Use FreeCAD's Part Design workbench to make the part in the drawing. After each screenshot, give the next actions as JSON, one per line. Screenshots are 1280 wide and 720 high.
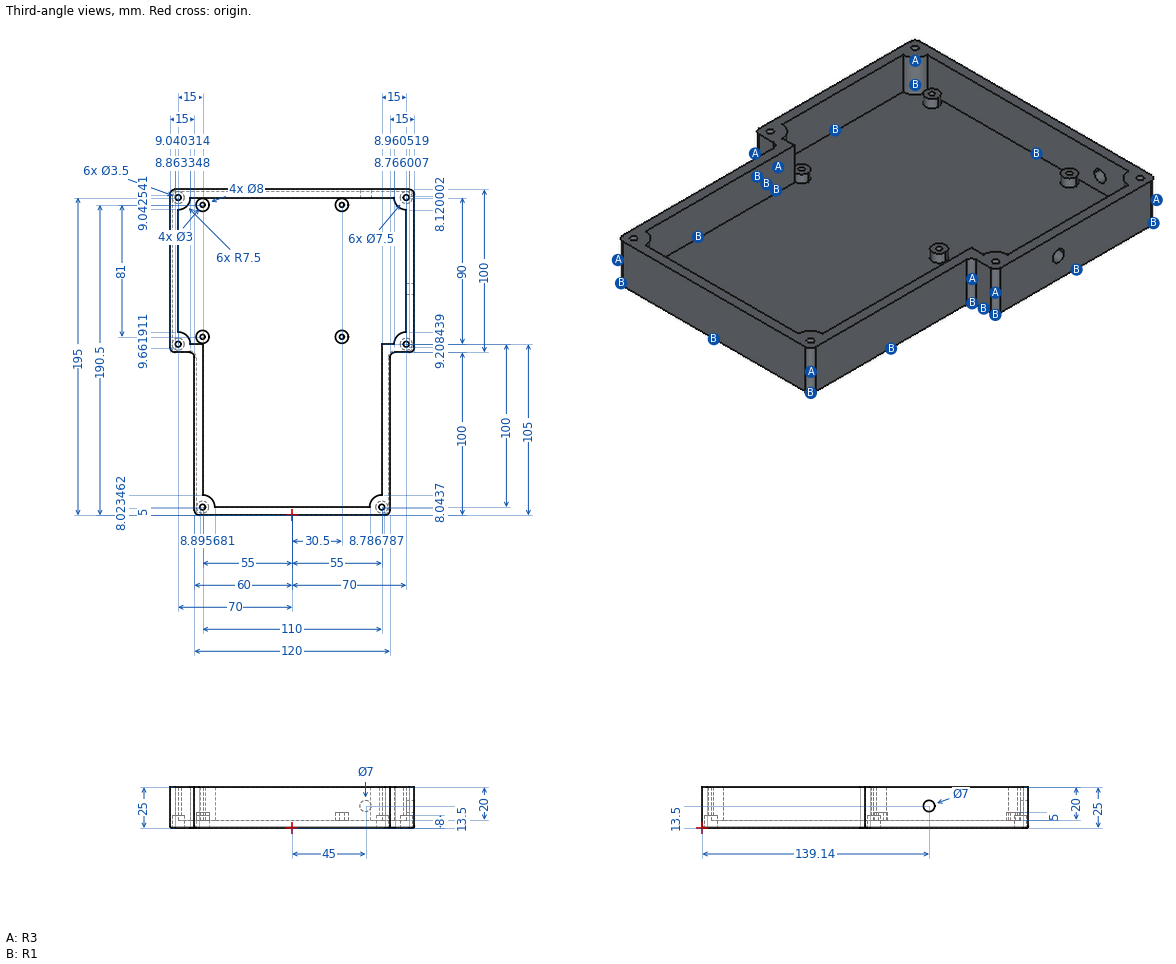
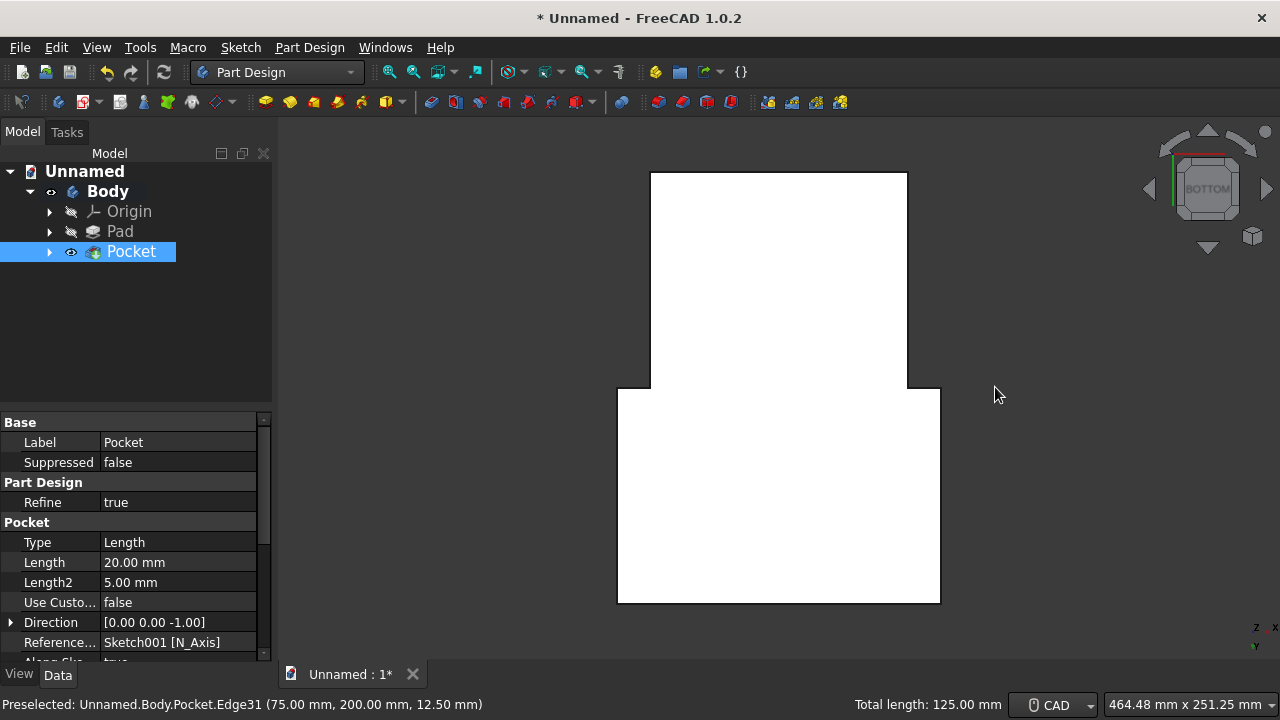
{"action": "key", "text": "4"}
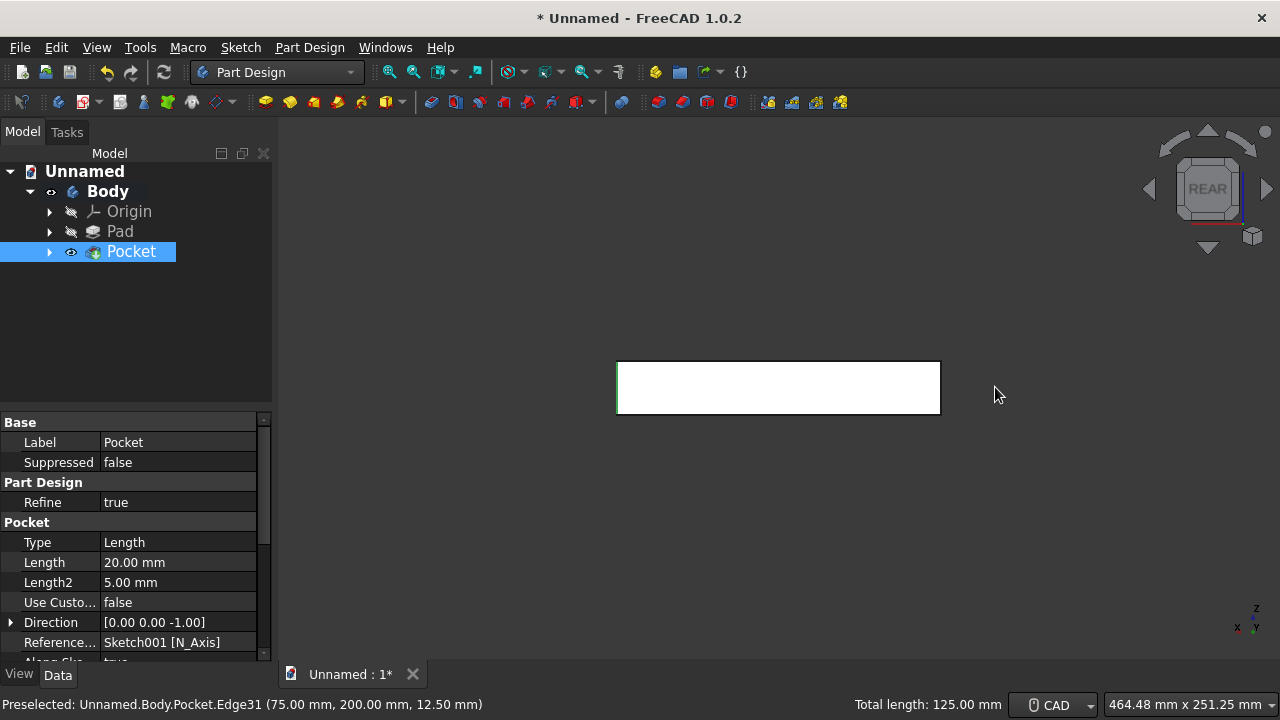
{"action": "key", "text": "v f"}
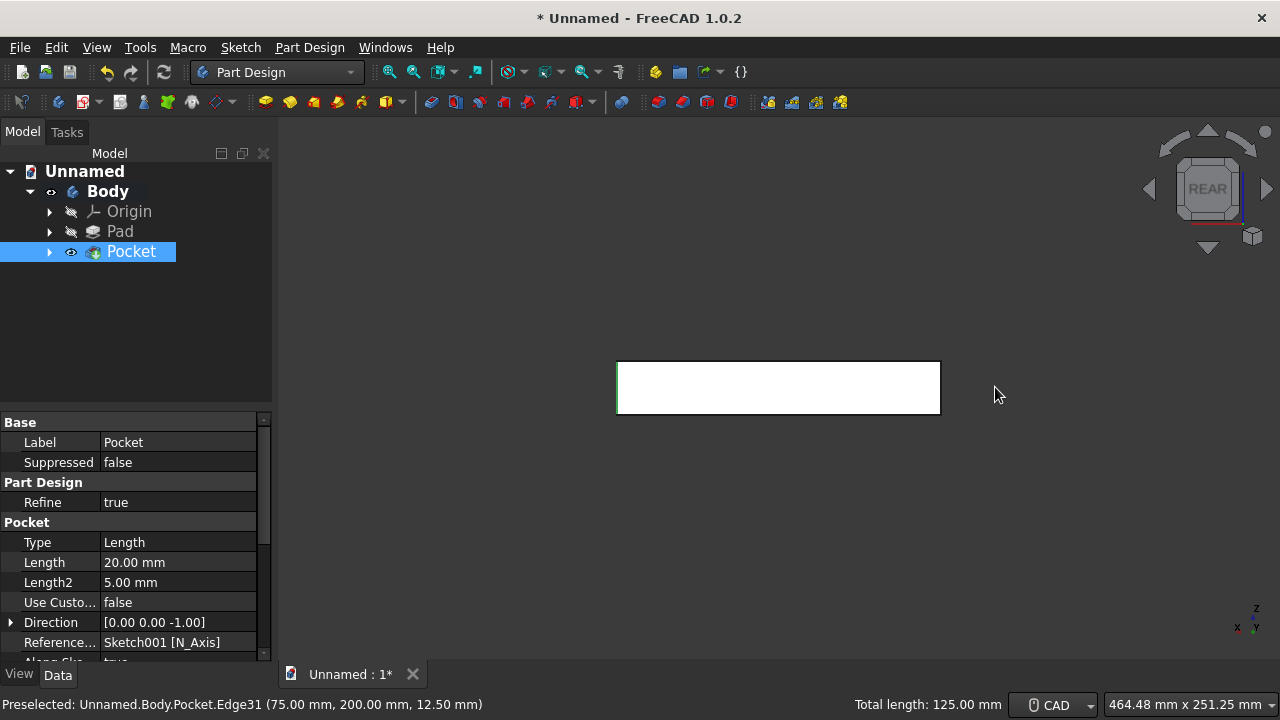
{"action": "left_click", "coordinate": [941, 387], "text": "ctrl"}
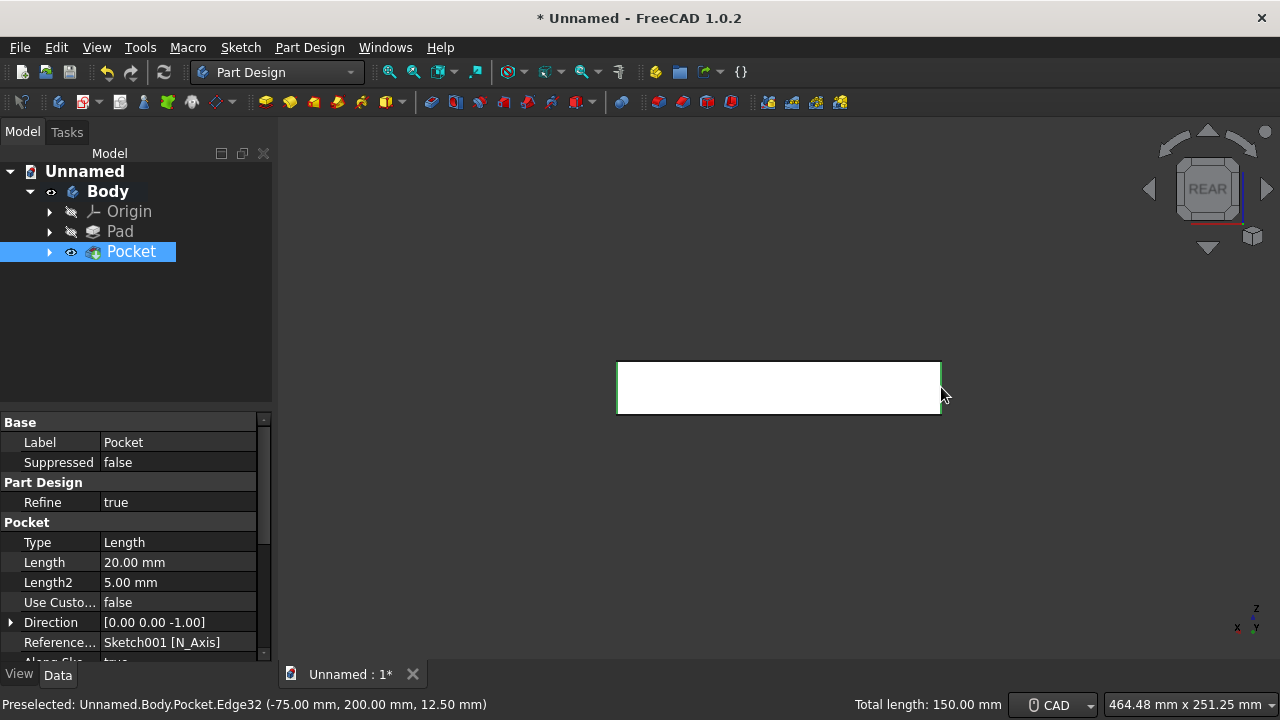
{"action": "key", "text": "6"}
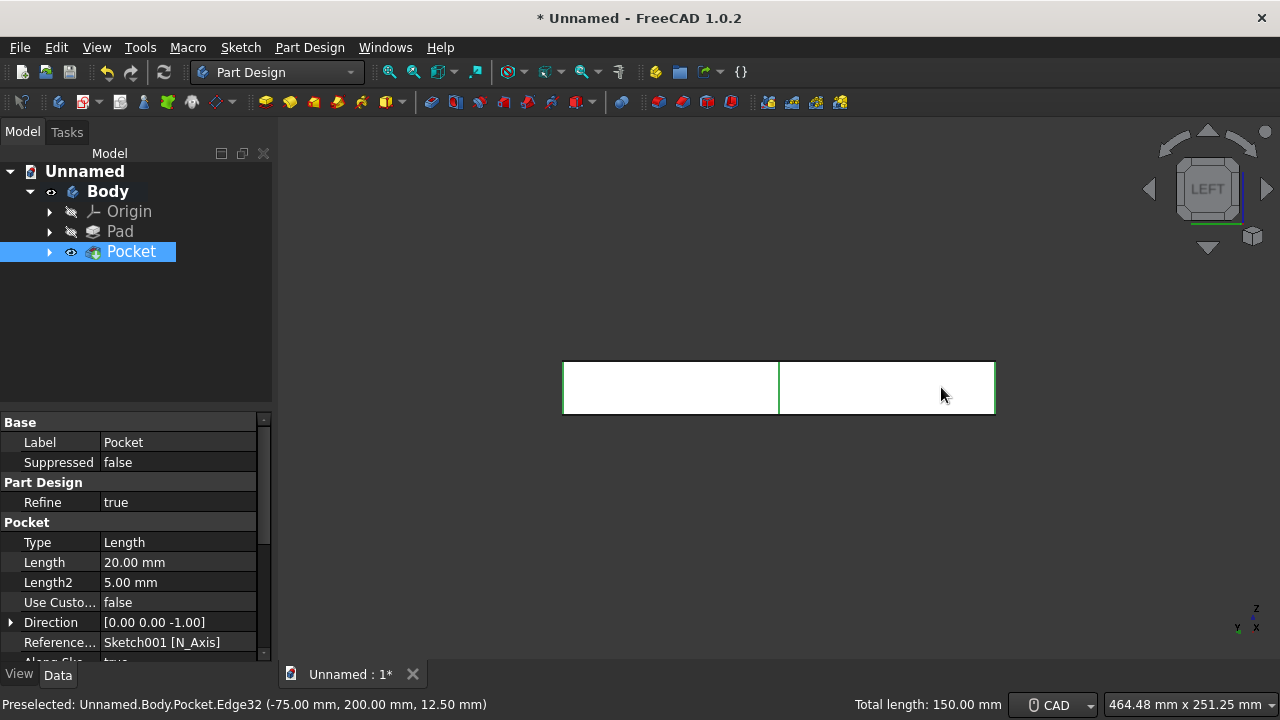
{"action": "key", "text": "v f"}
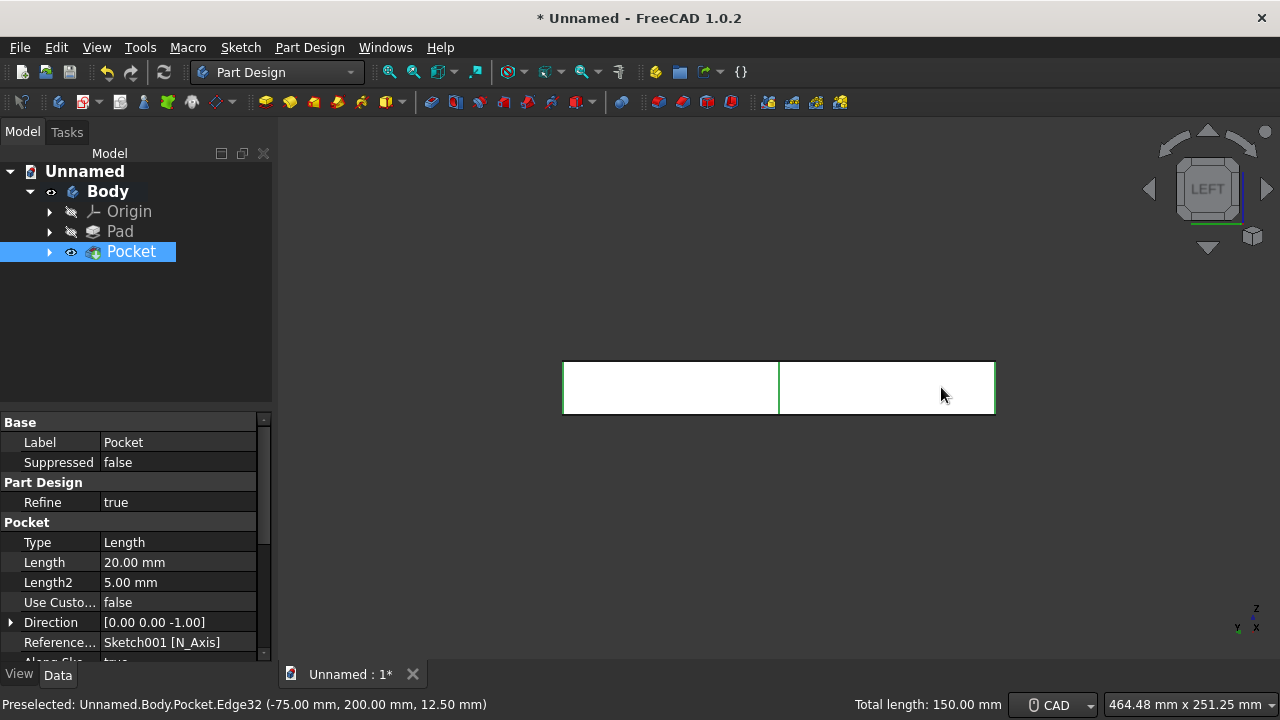
{"action": "key", "text": "v 3"}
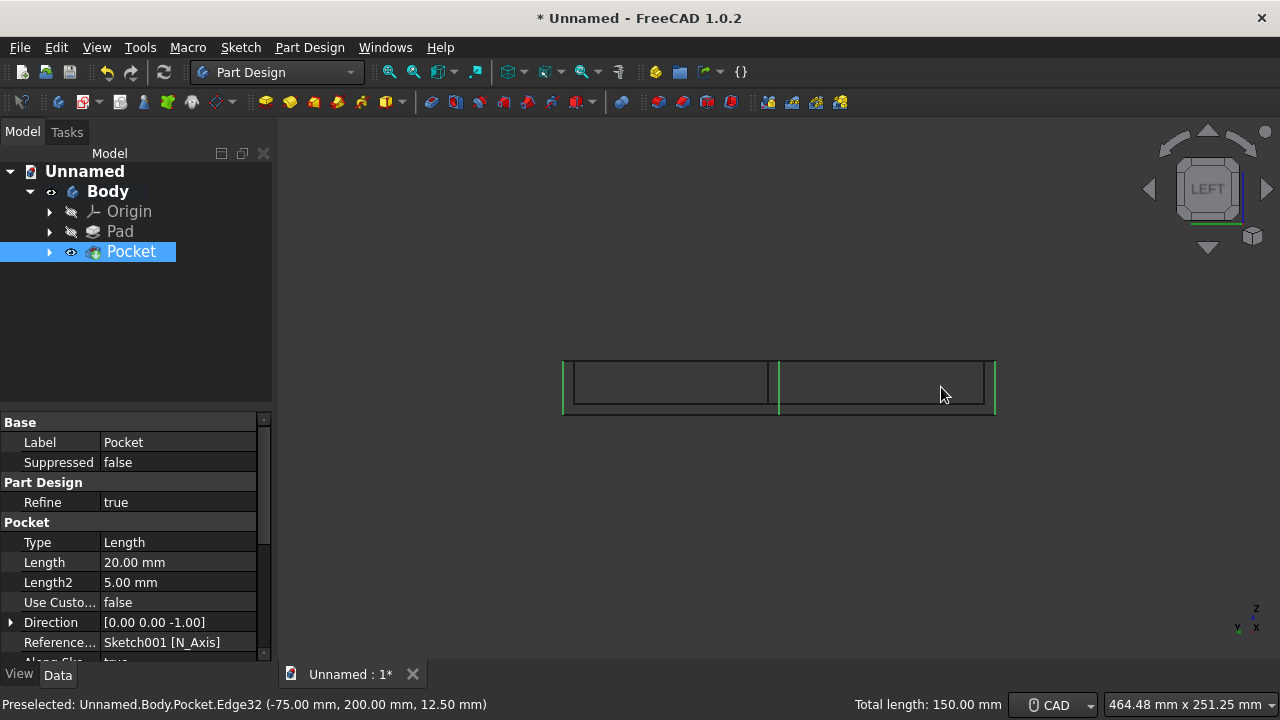
{"action": "key", "text": "0"}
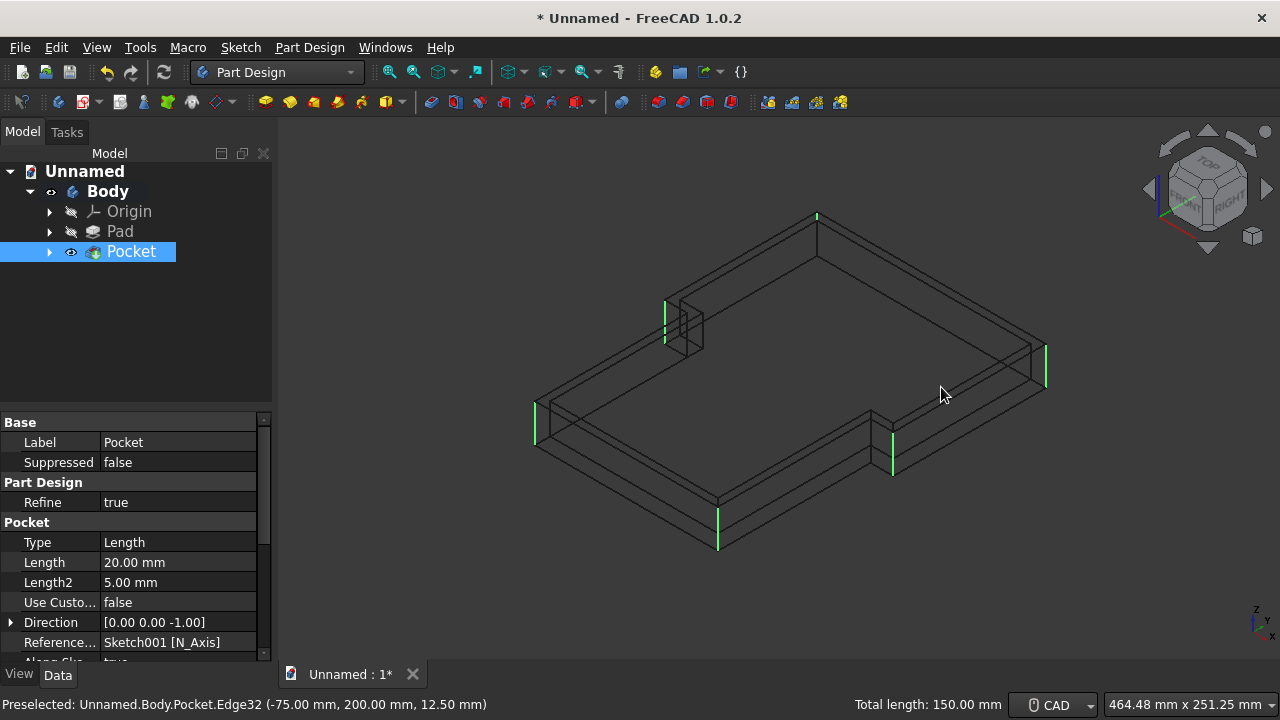
{"action": "left_click", "coordinate": [871, 440], "text": "ctrl"}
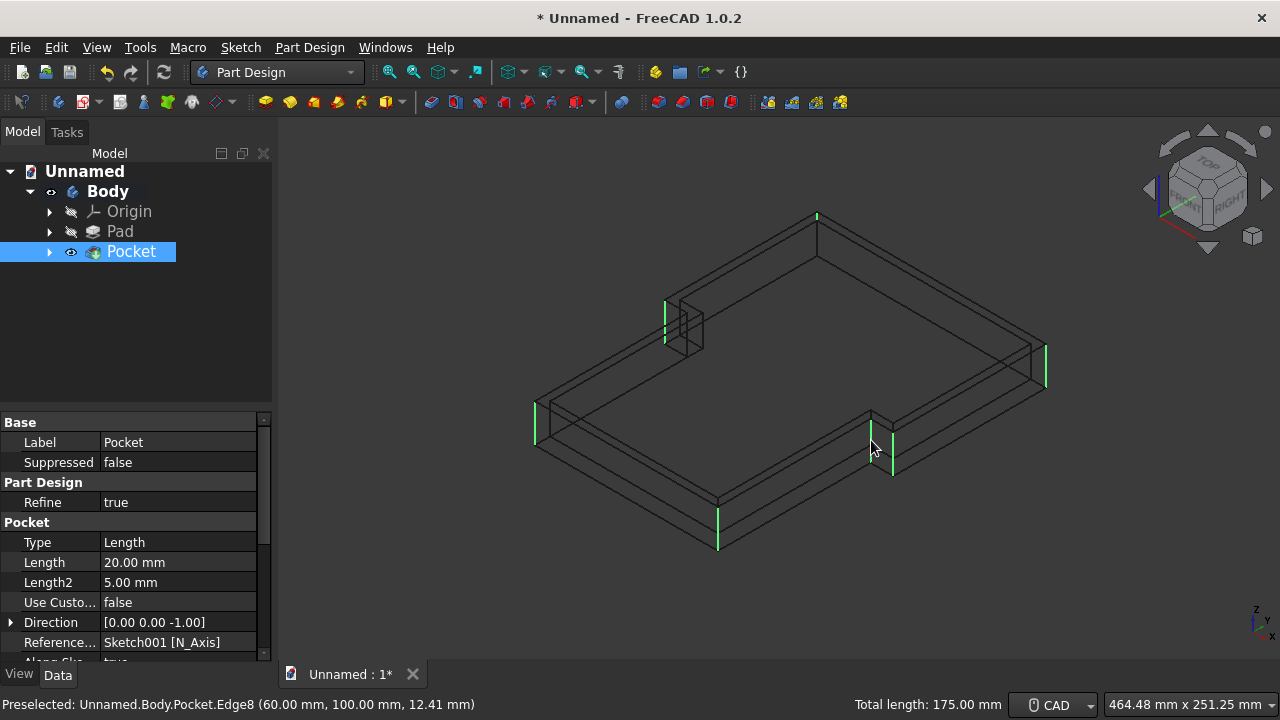
{"action": "left_click", "coordinate": [687, 334], "text": "ctrl"}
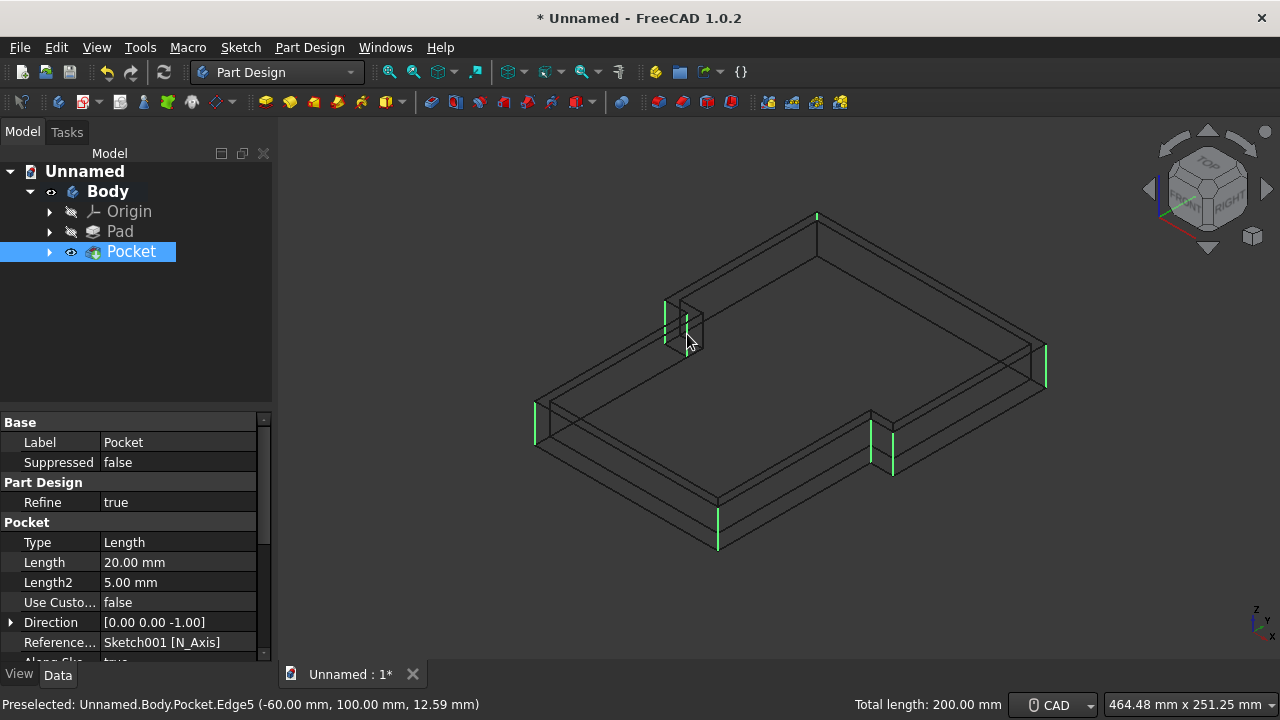
{"action": "key", "text": "v 1"}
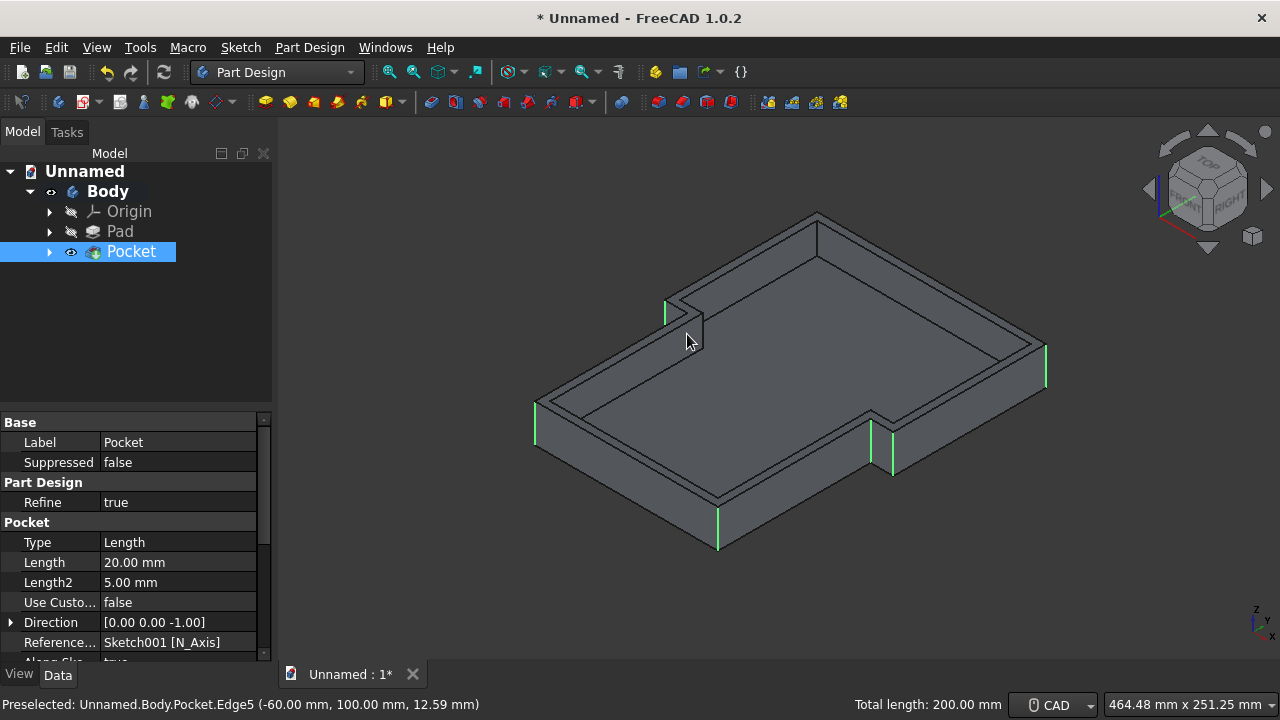
{"action": "left_click", "coordinate": [660, 102]}